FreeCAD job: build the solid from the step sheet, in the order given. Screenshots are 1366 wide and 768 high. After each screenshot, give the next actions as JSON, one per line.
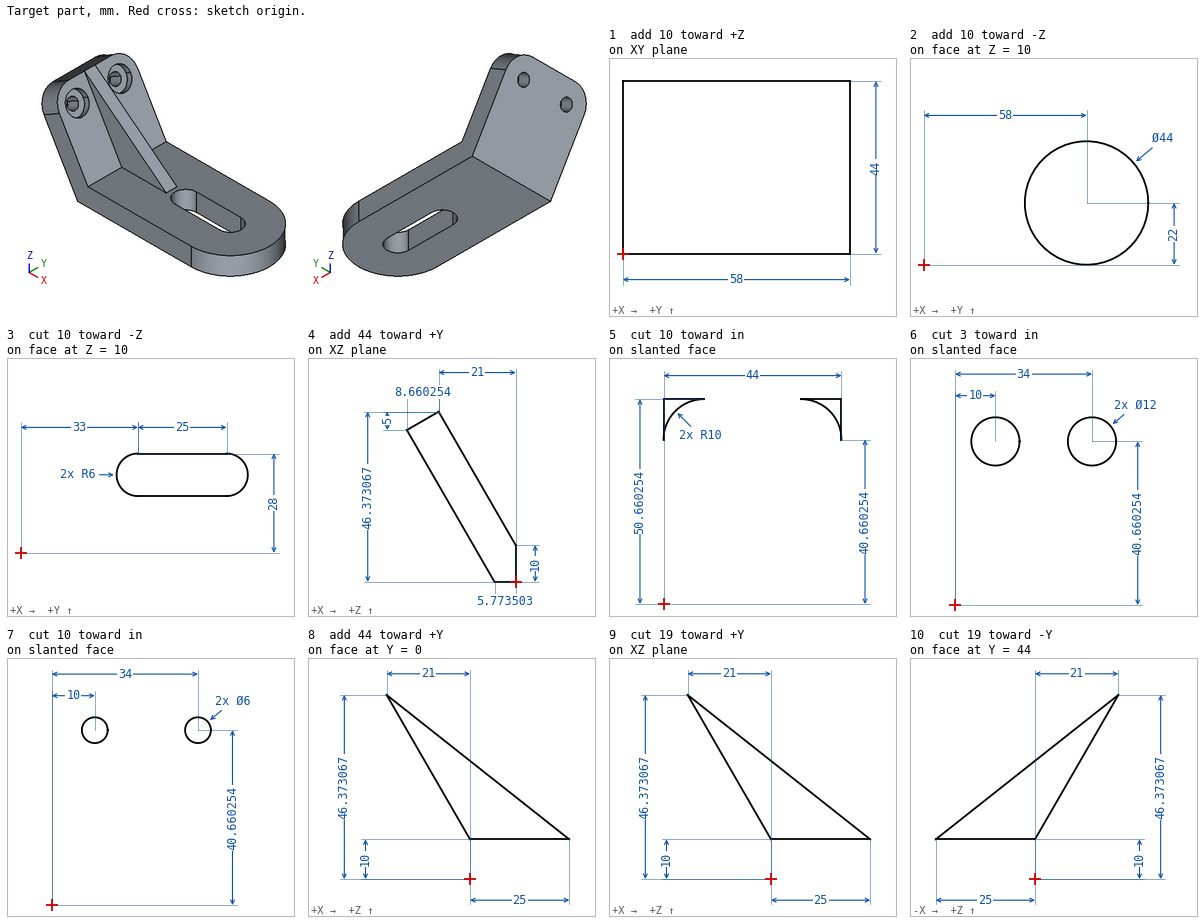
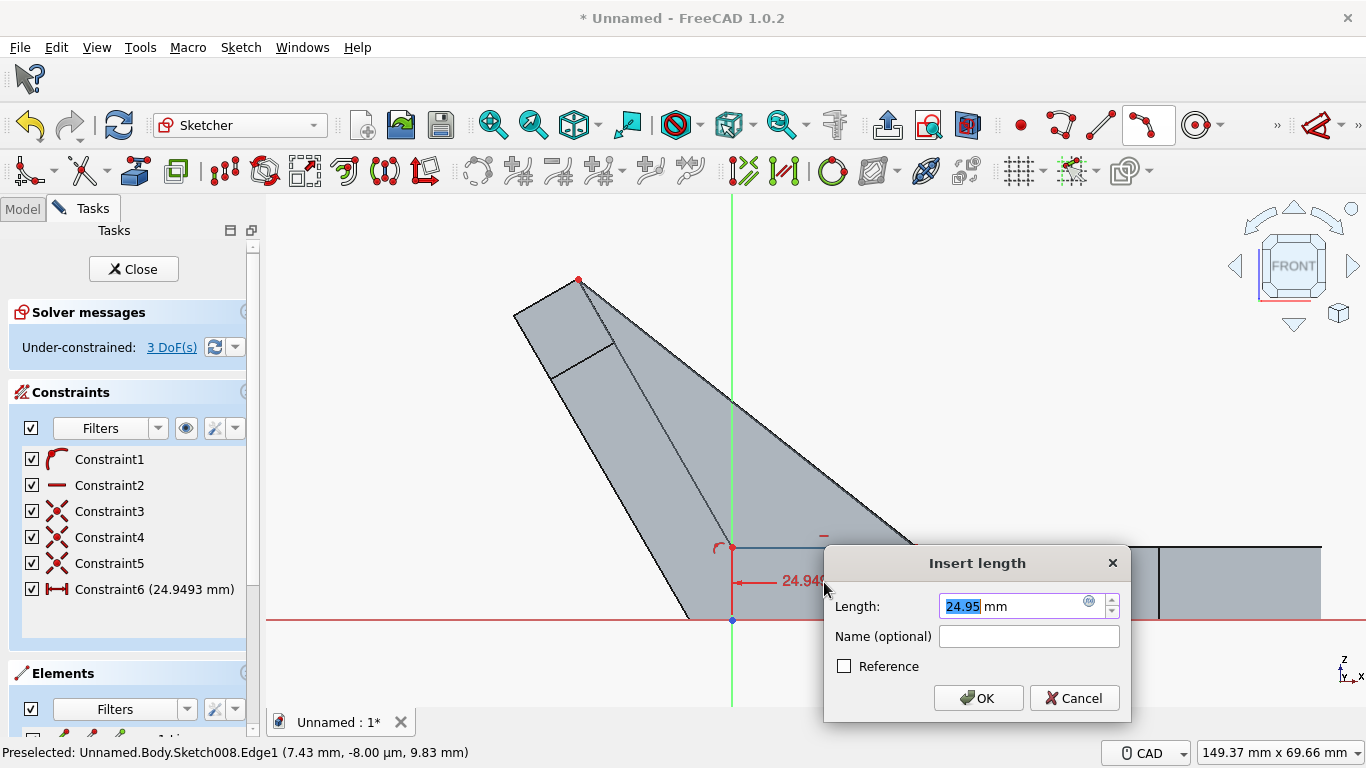
{"action": "type", "text": "25"}
{"action": "key", "text": "Return"}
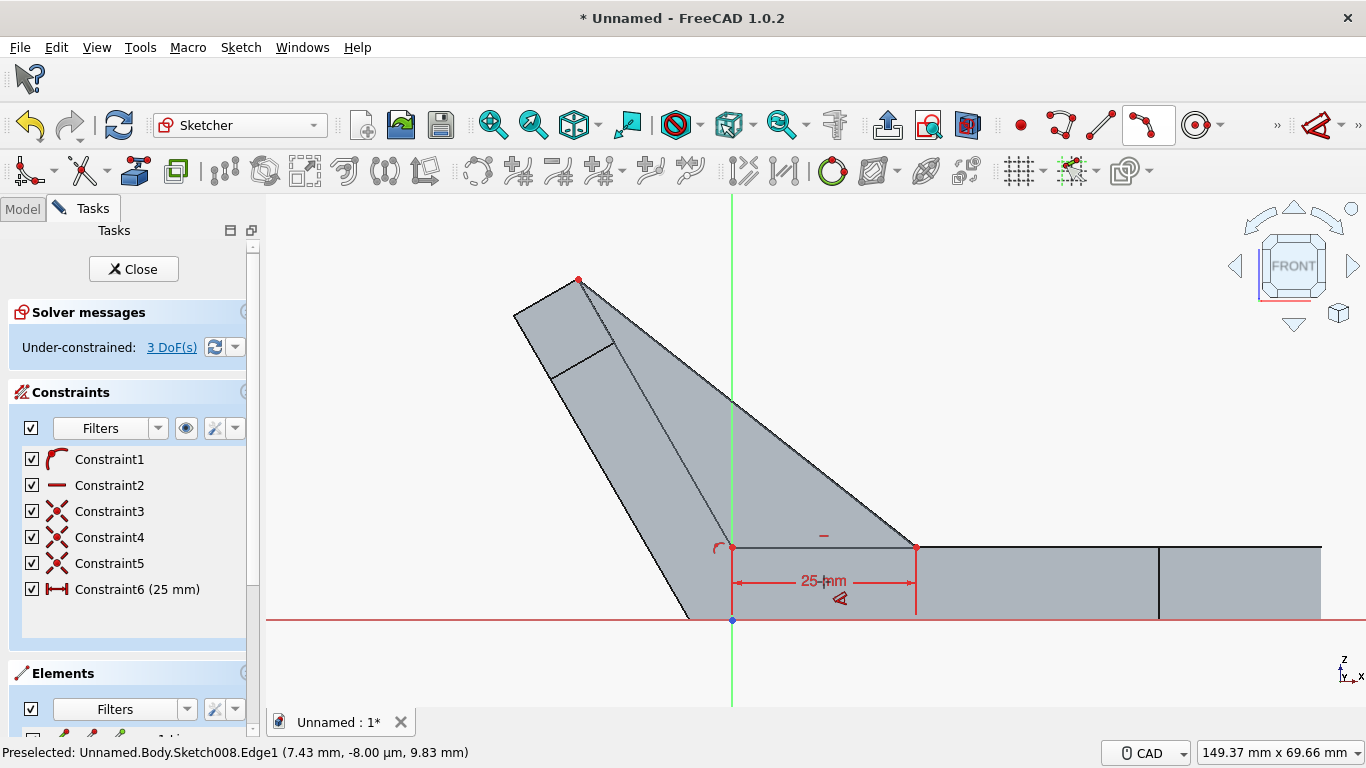
{"action": "left_click", "coordinate": [732, 548]}
{"action": "left_click", "coordinate": [698, 584]}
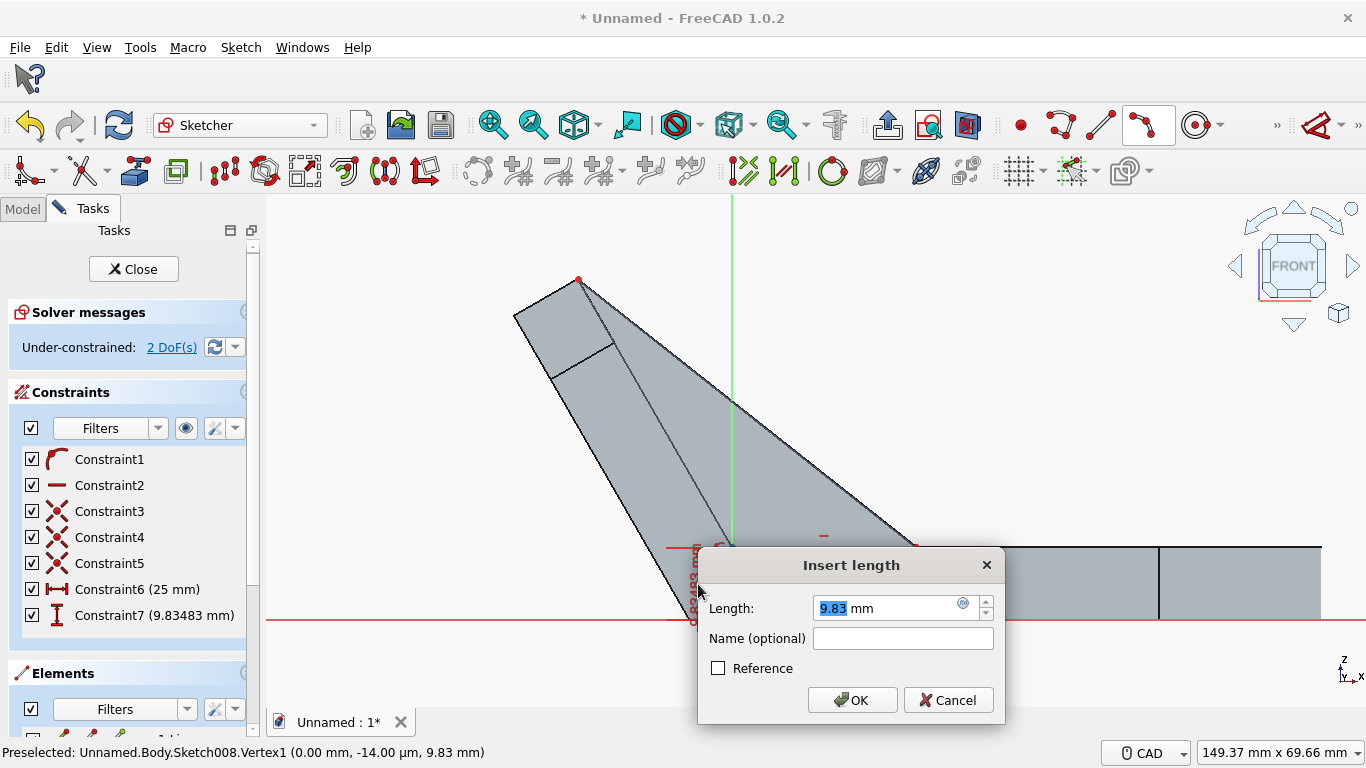
{"action": "type", "text": "10"}
{"action": "key", "text": "Return"}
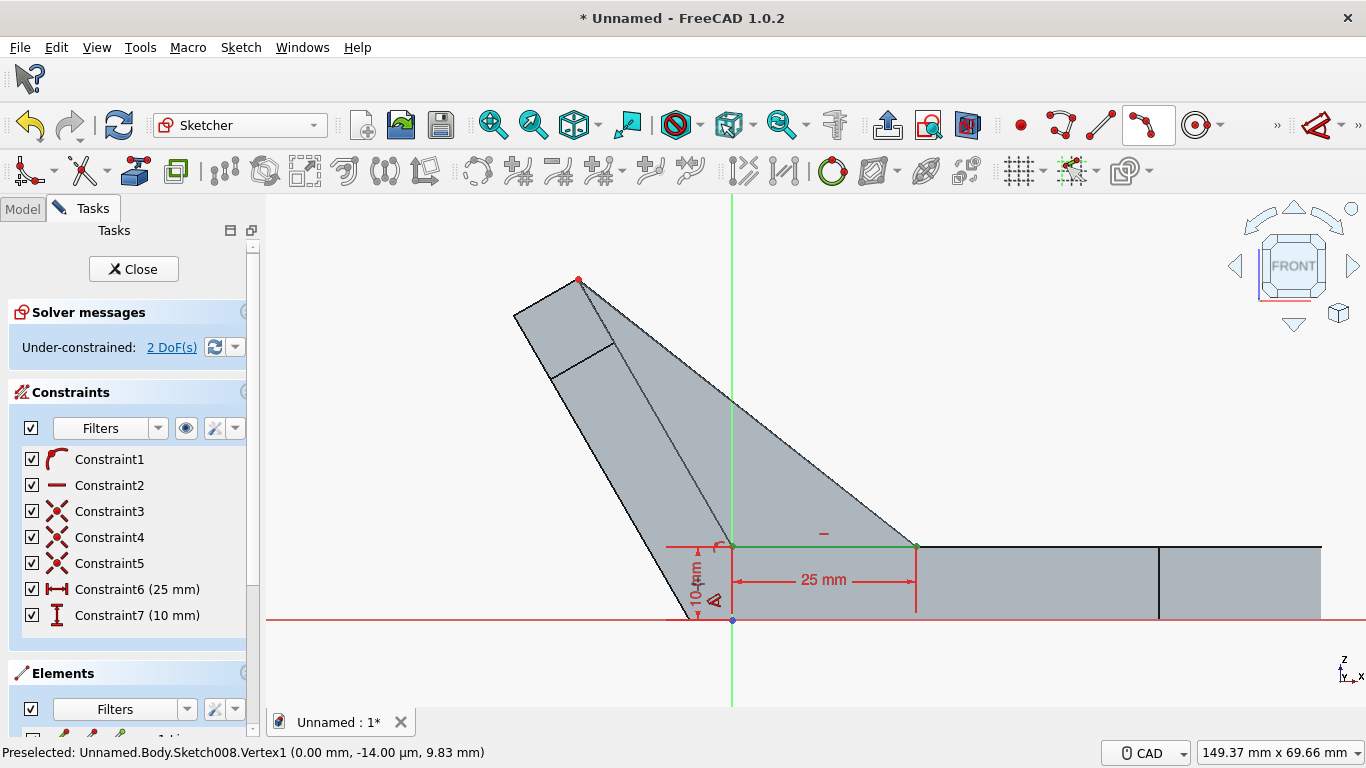
{"action": "left_click", "coordinate": [578, 280]}
{"action": "left_click", "coordinate": [655, 654]}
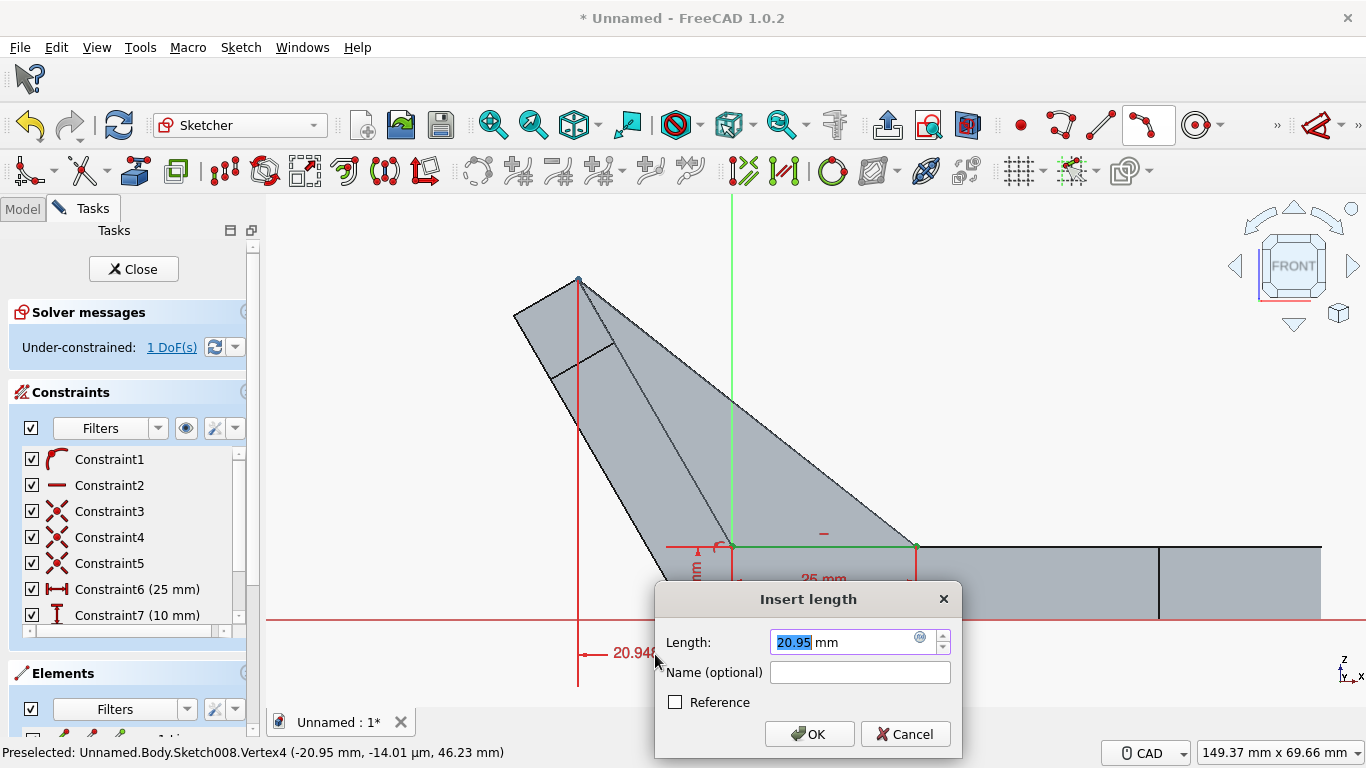
{"action": "type", "text": "21"}
{"action": "key", "text": "Return"}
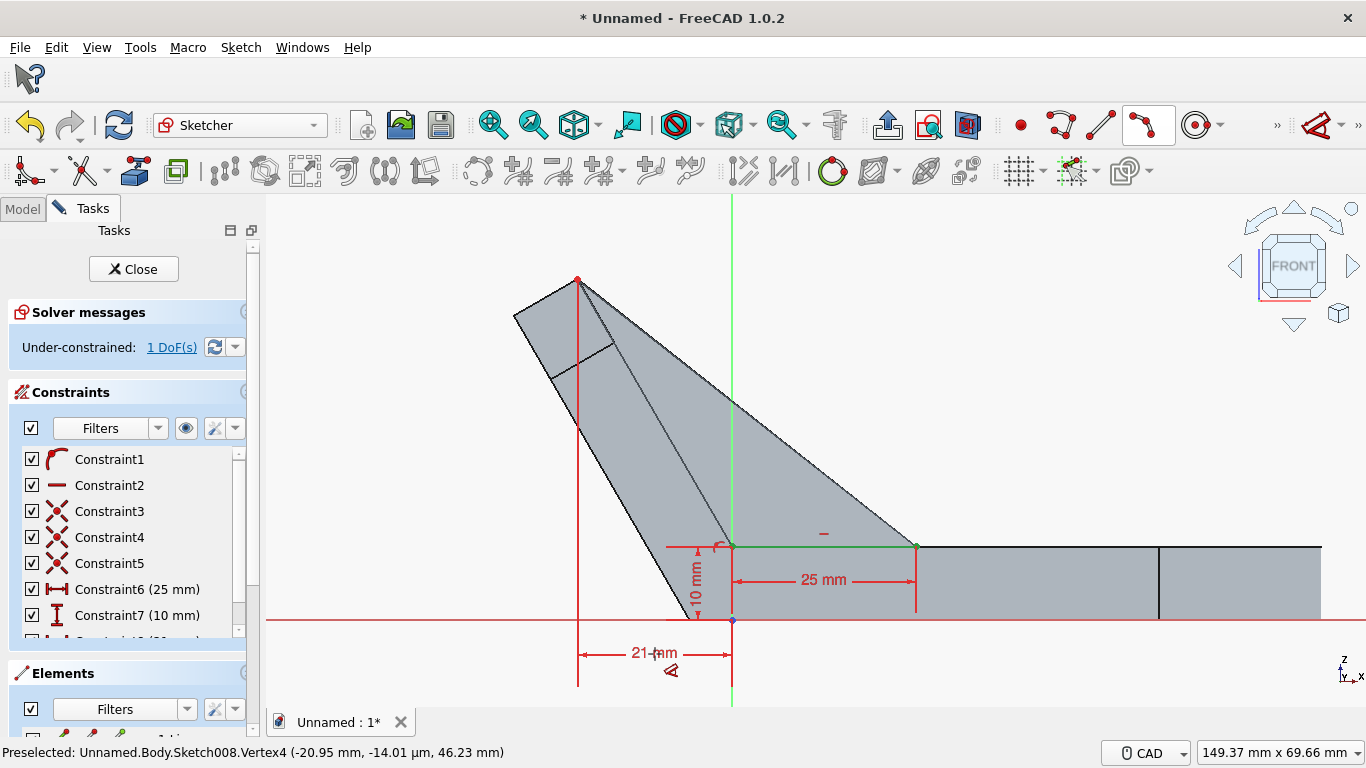
{"action": "left_click", "coordinate": [578, 280]}
{"action": "left_click", "coordinate": [544, 450]}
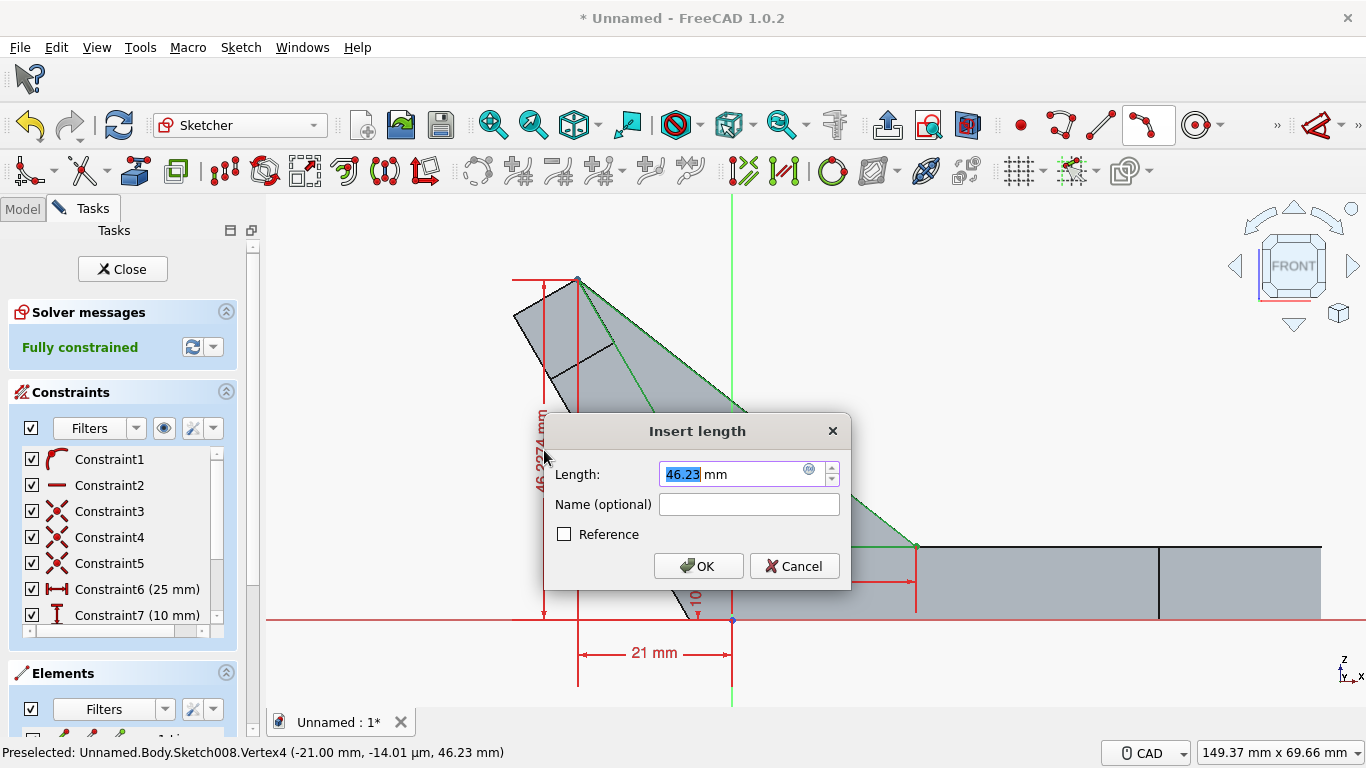
{"action": "type", "text": "46.373067"}
{"action": "key", "text": "Return"}
{"action": "key", "text": "Escape"}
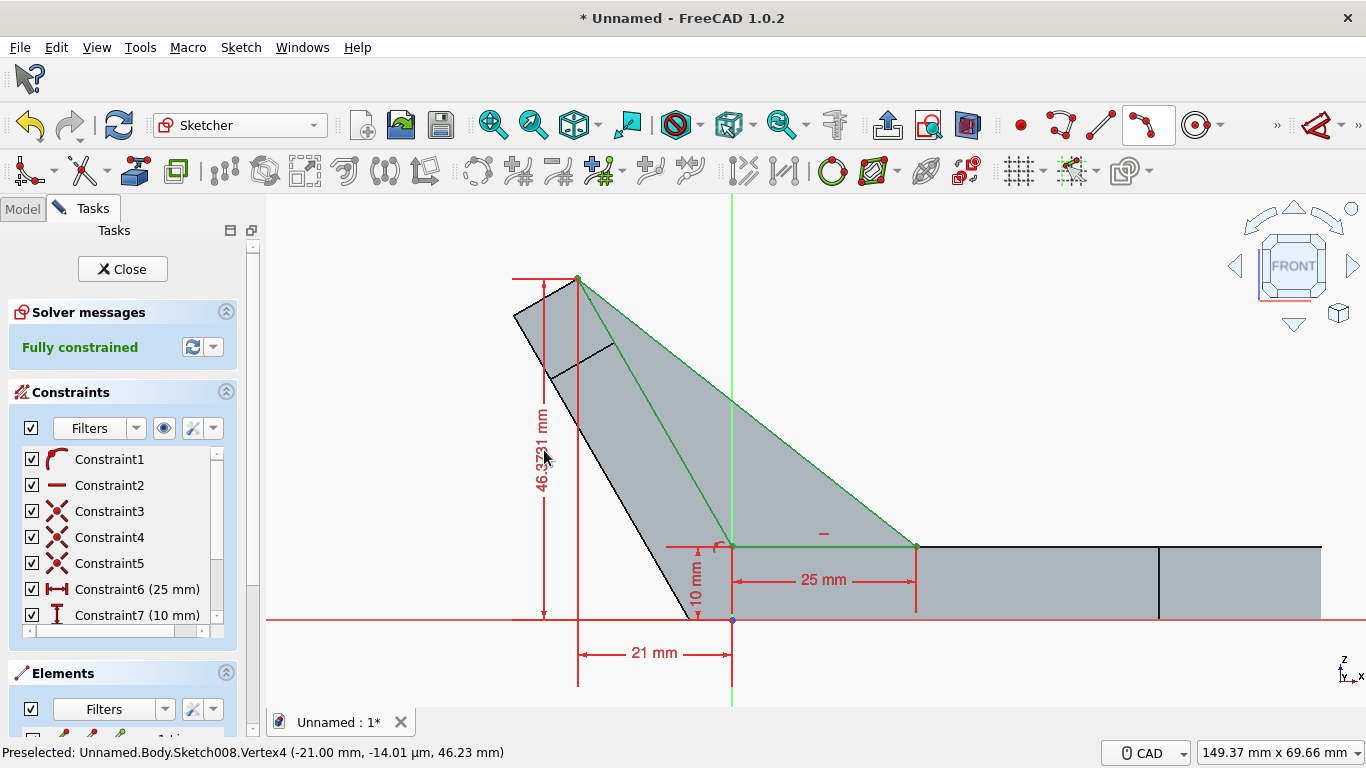
{"action": "left_click", "coordinate": [123, 269]}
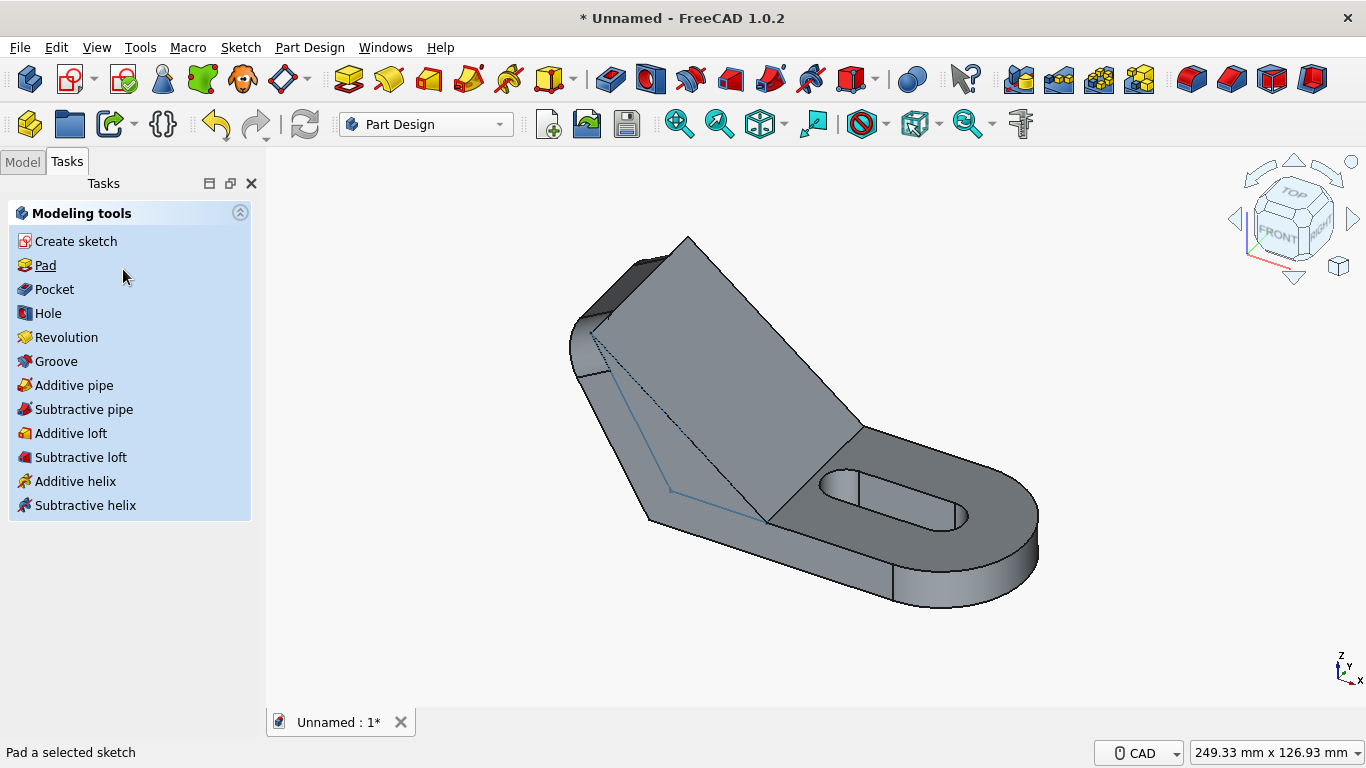
{"action": "left_click", "coordinate": [612, 80]}